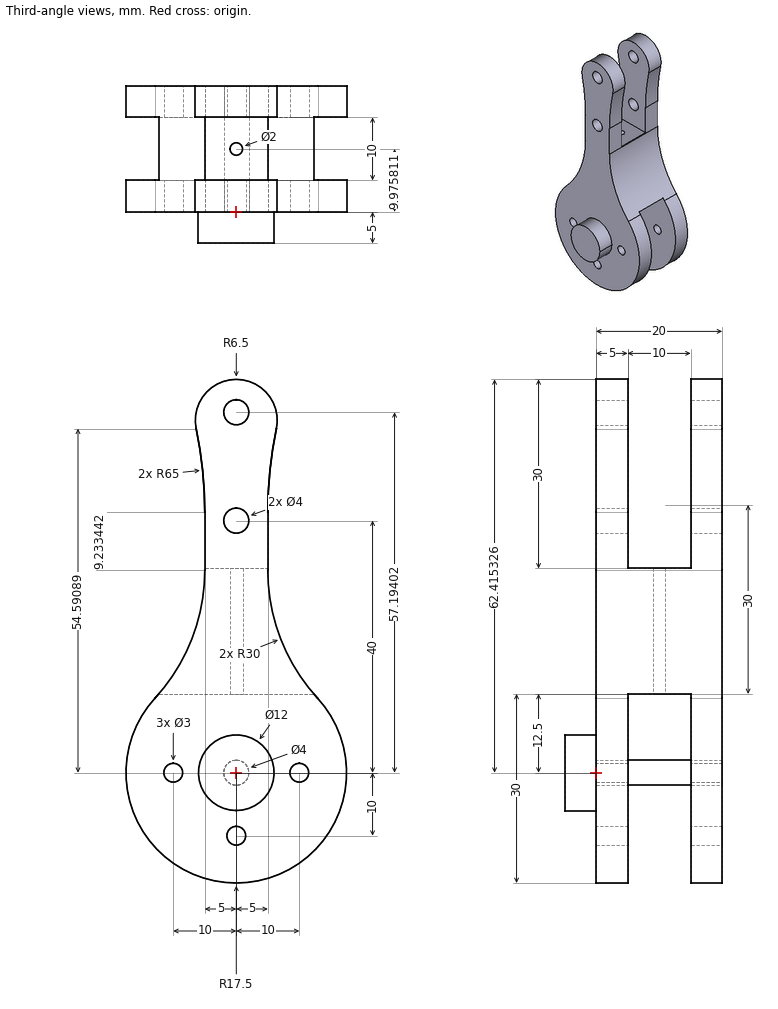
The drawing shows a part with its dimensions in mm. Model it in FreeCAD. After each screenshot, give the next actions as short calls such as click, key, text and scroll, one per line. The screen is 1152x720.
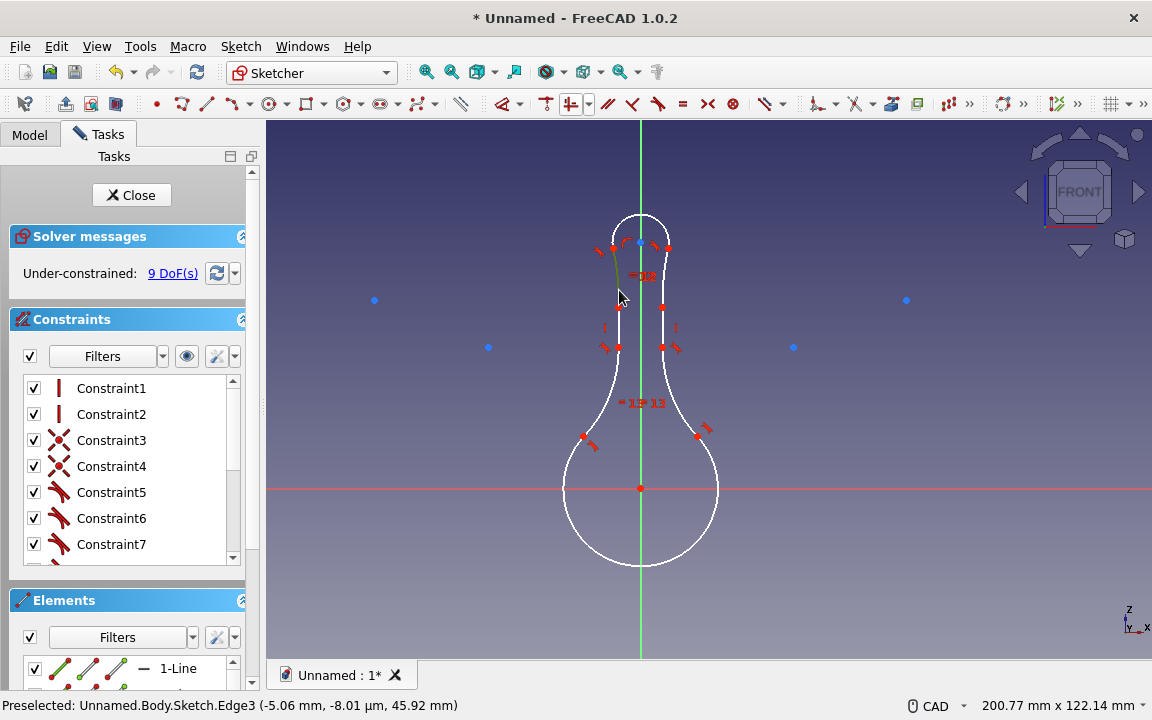
key(k)
key(r)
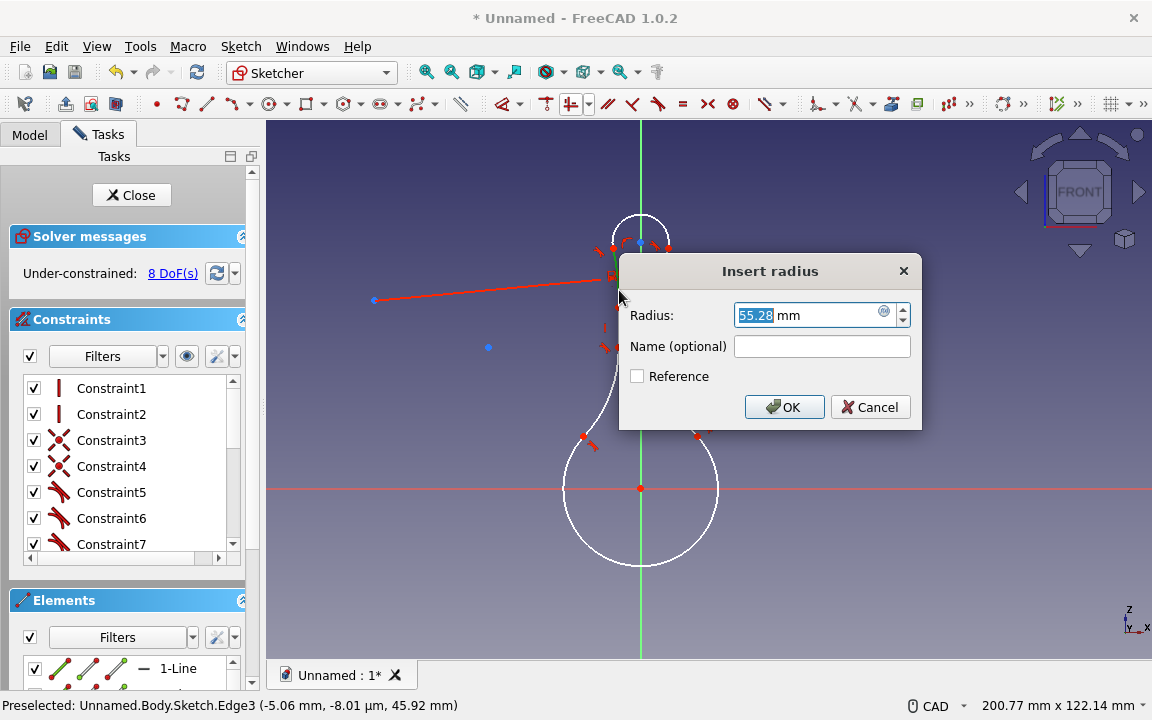
text(65)
key(Return)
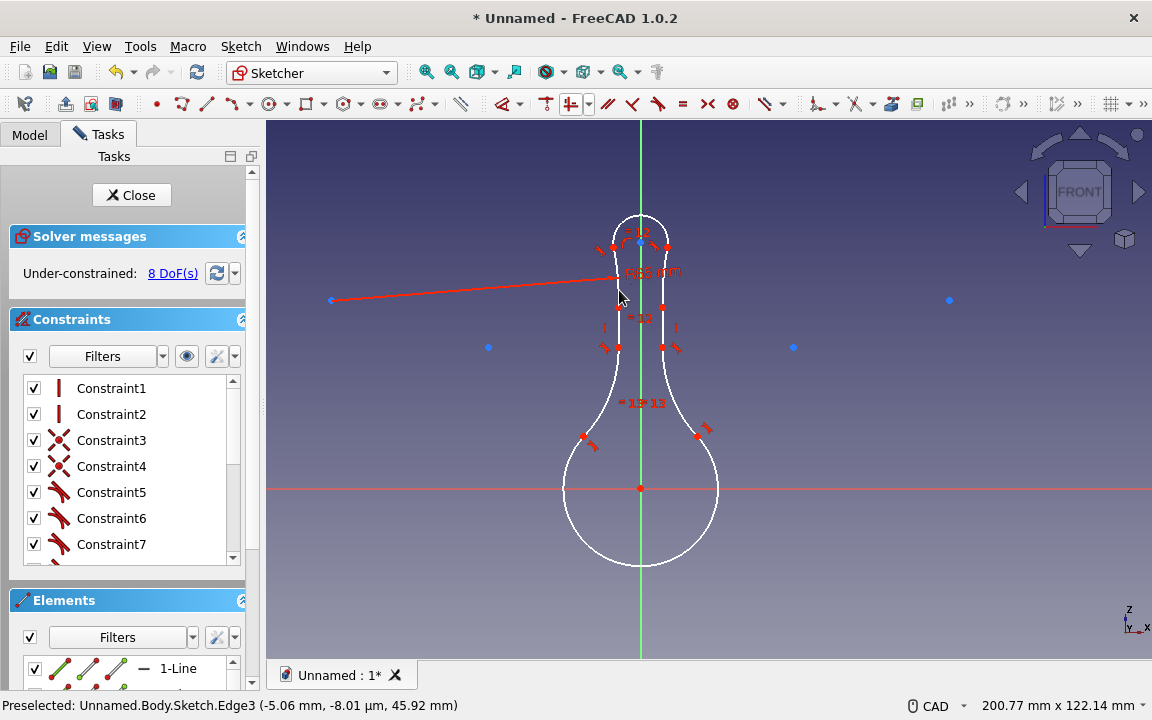
scroll(658, 222, up, 2)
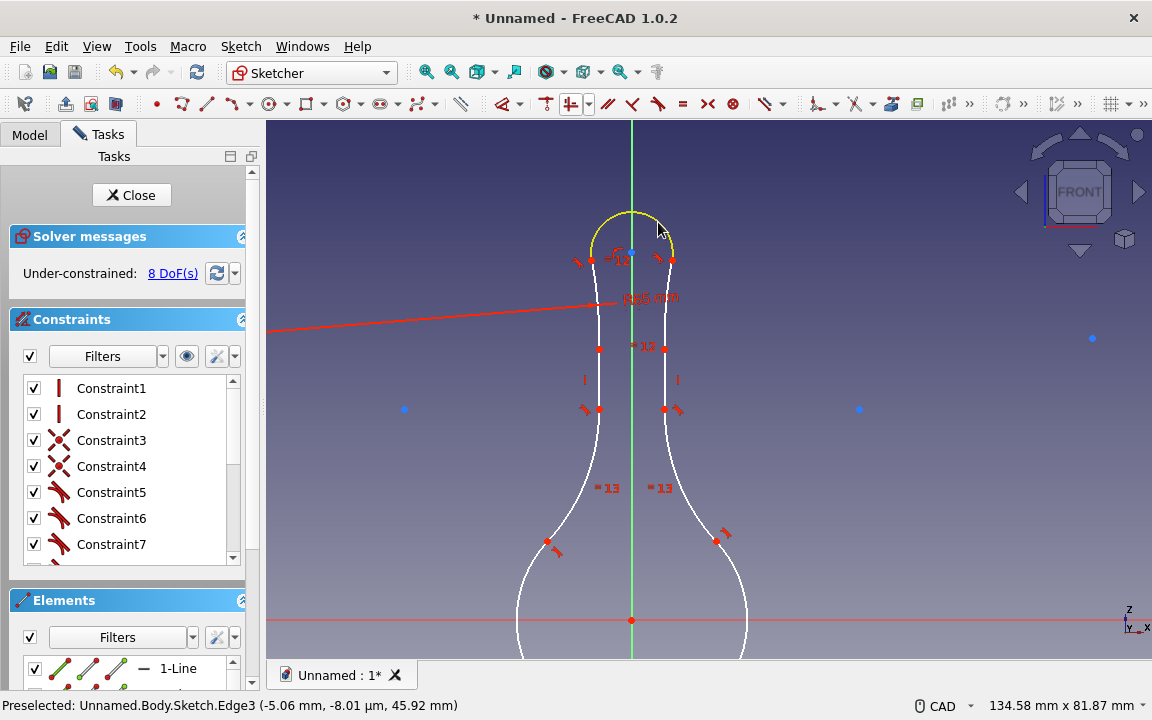
click(658, 222)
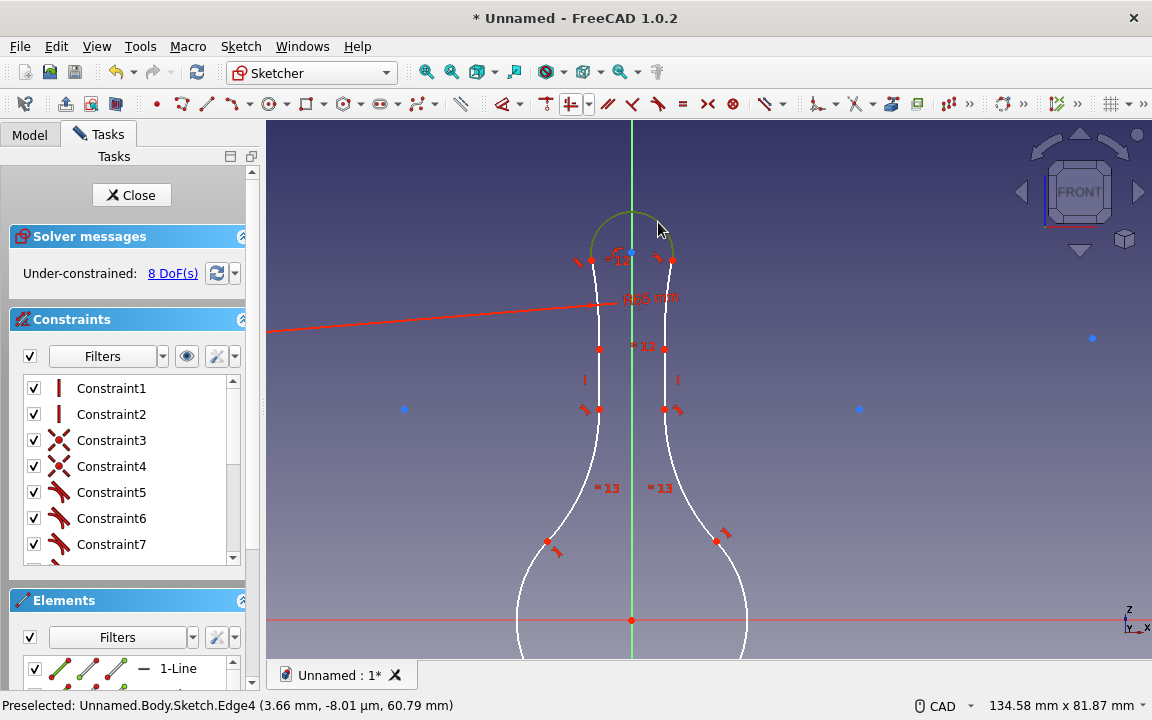
click(520, 104)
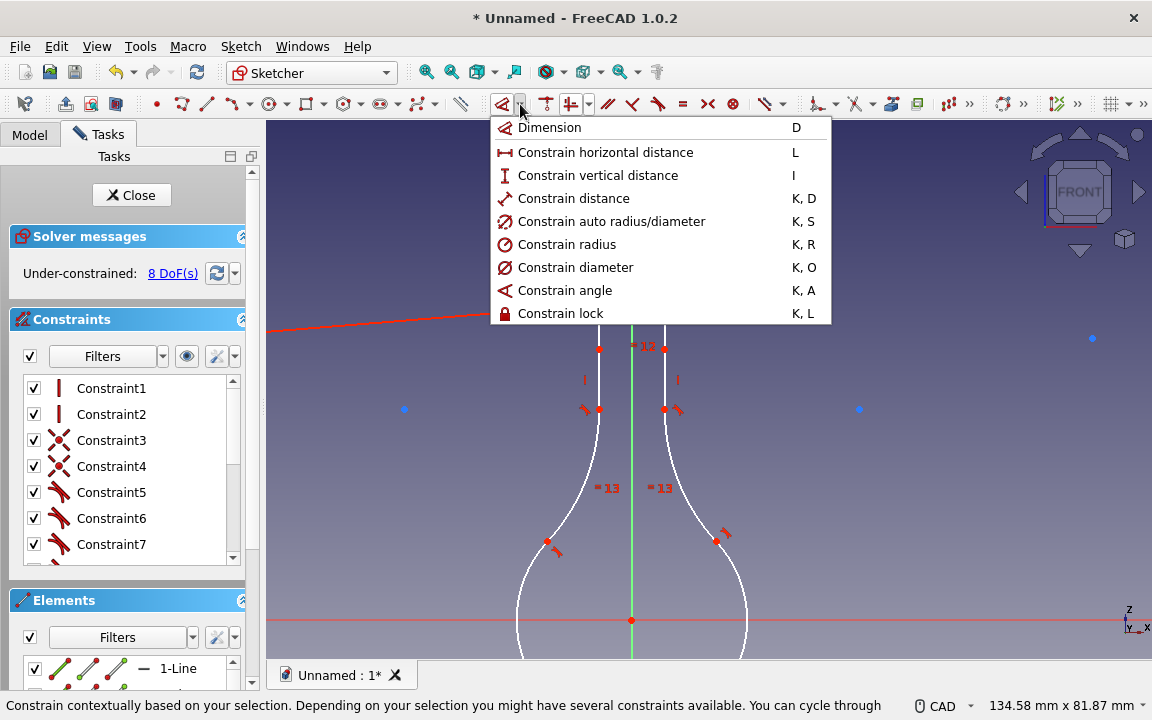
click(661, 244)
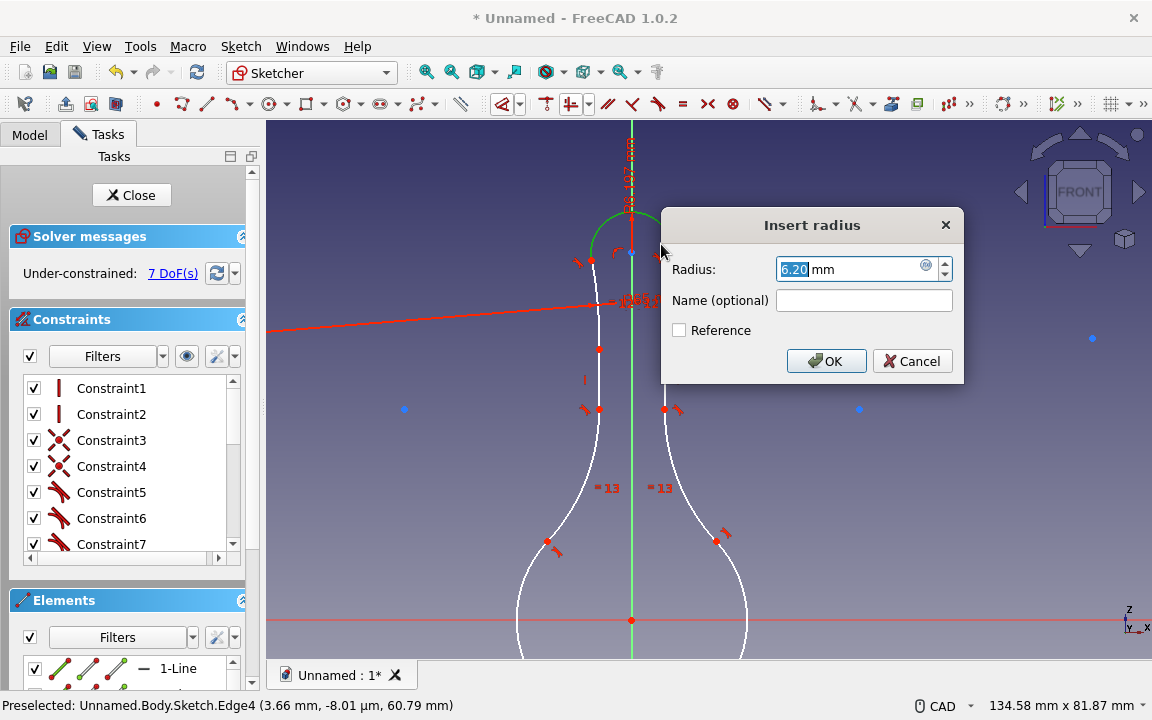
text(6.5)
key(Return)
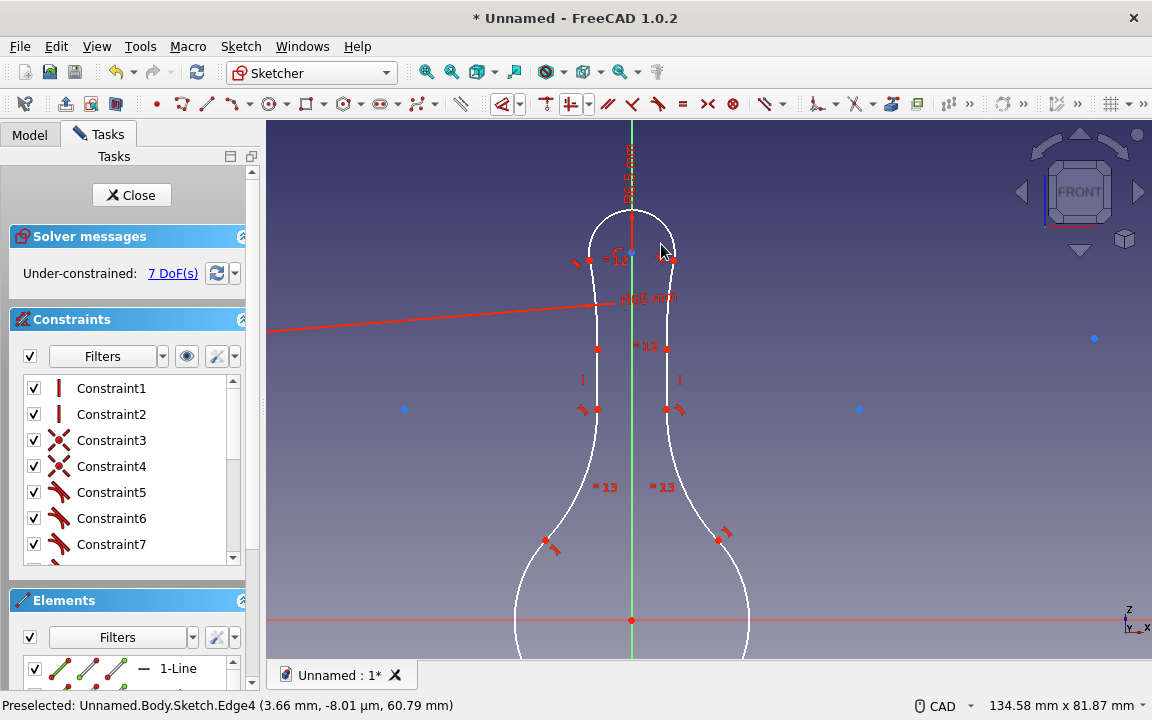
click(672, 453)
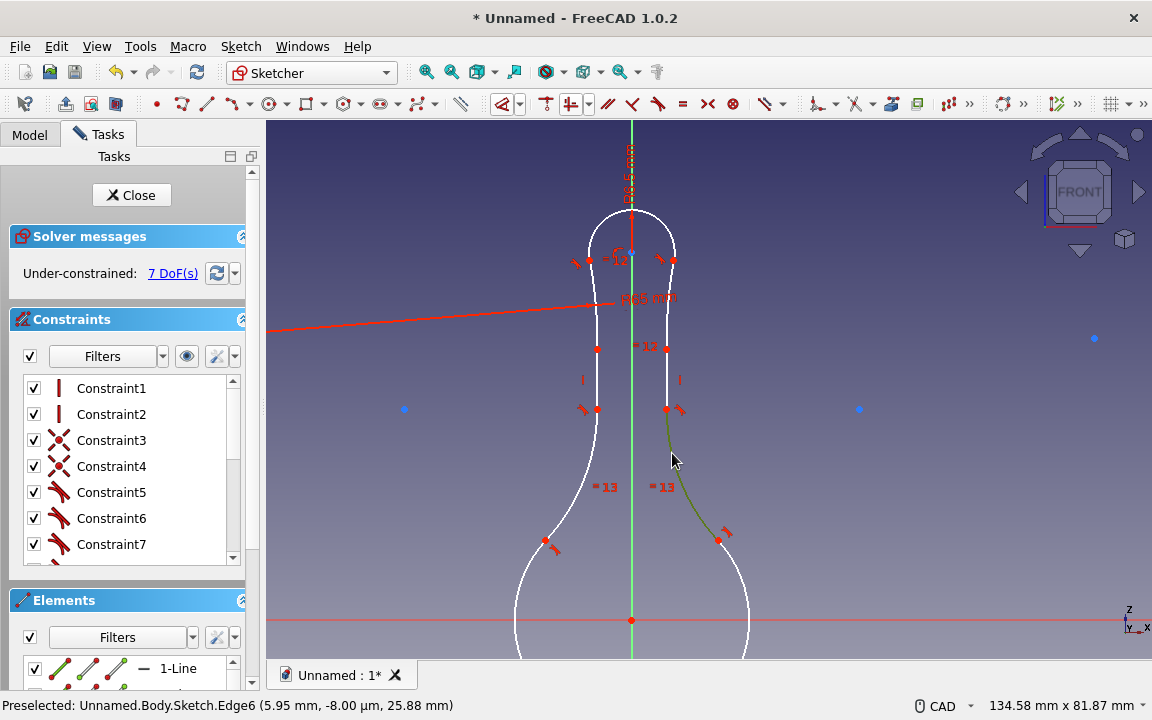
key(k)
key(r)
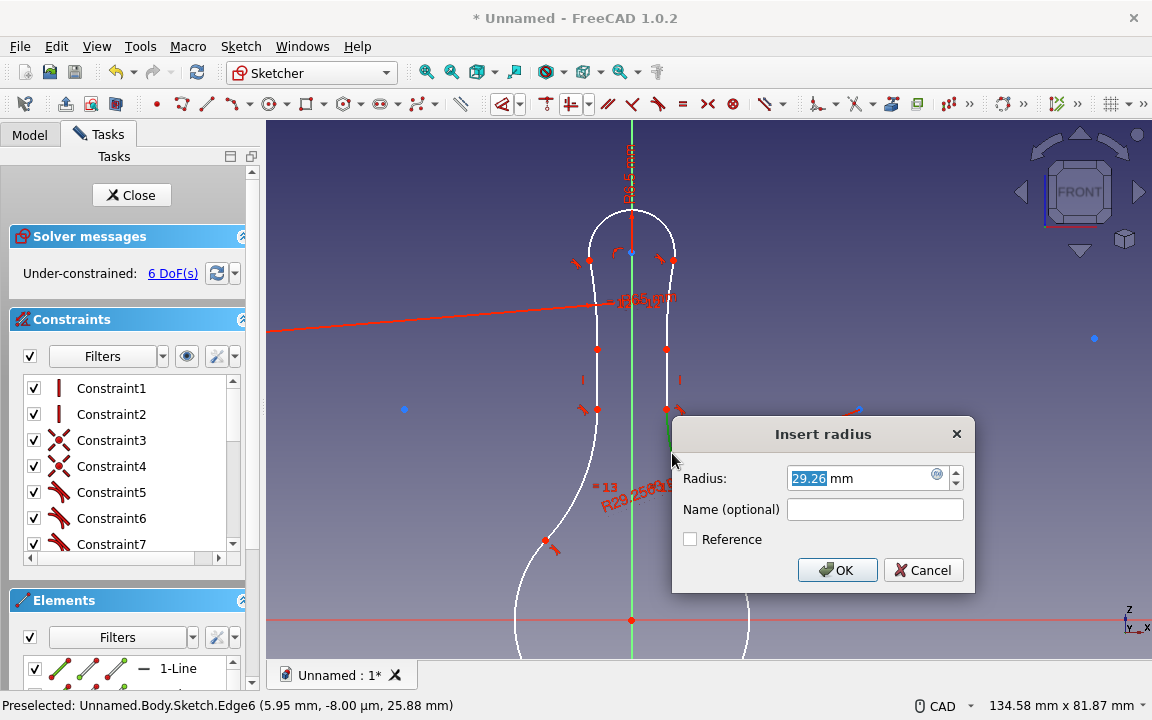
text(30)
key(Return)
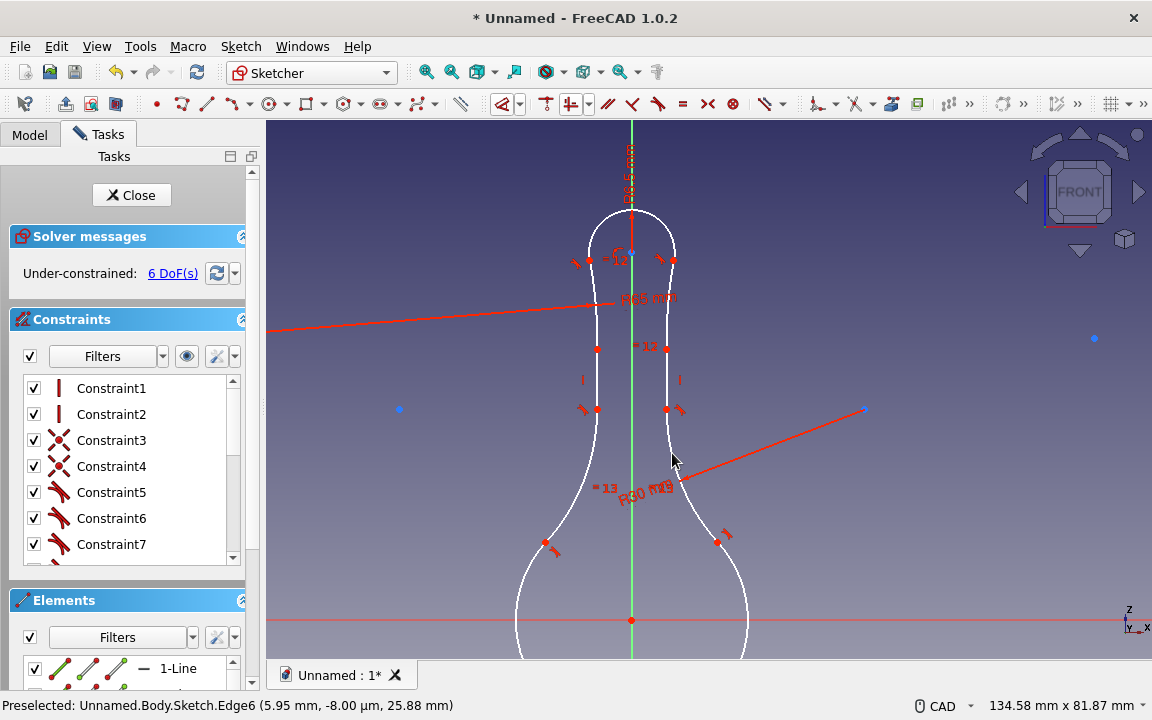
scroll(658, 221, down, 2)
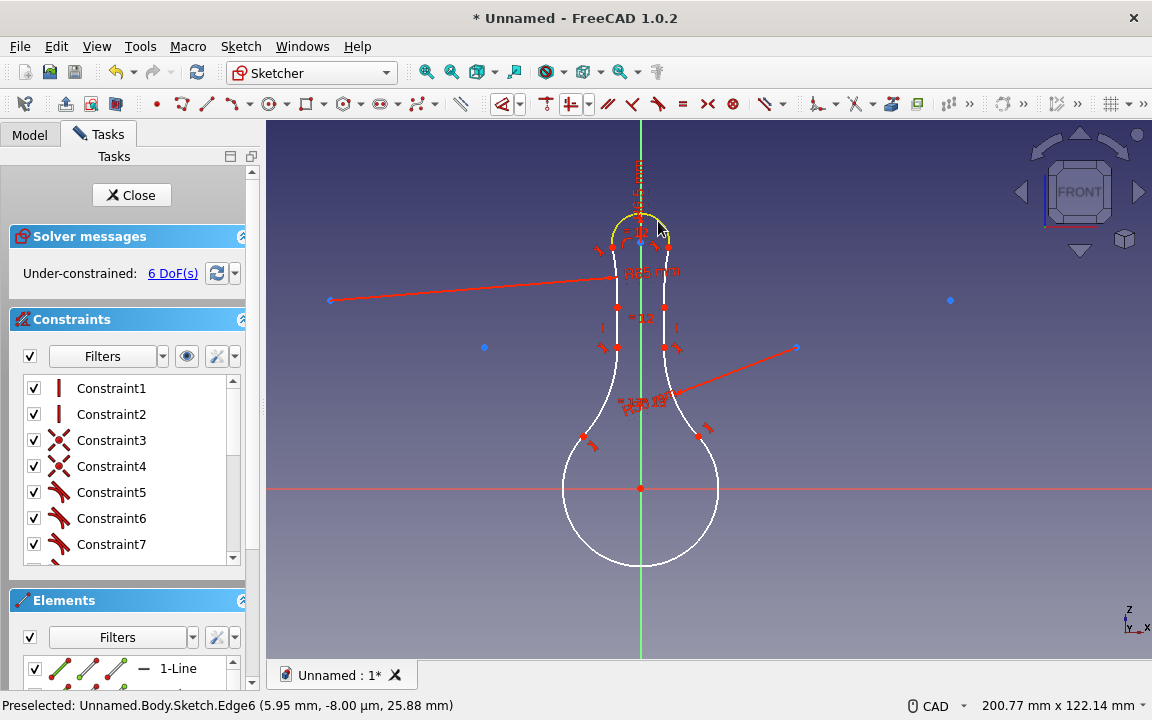
click(579, 536)